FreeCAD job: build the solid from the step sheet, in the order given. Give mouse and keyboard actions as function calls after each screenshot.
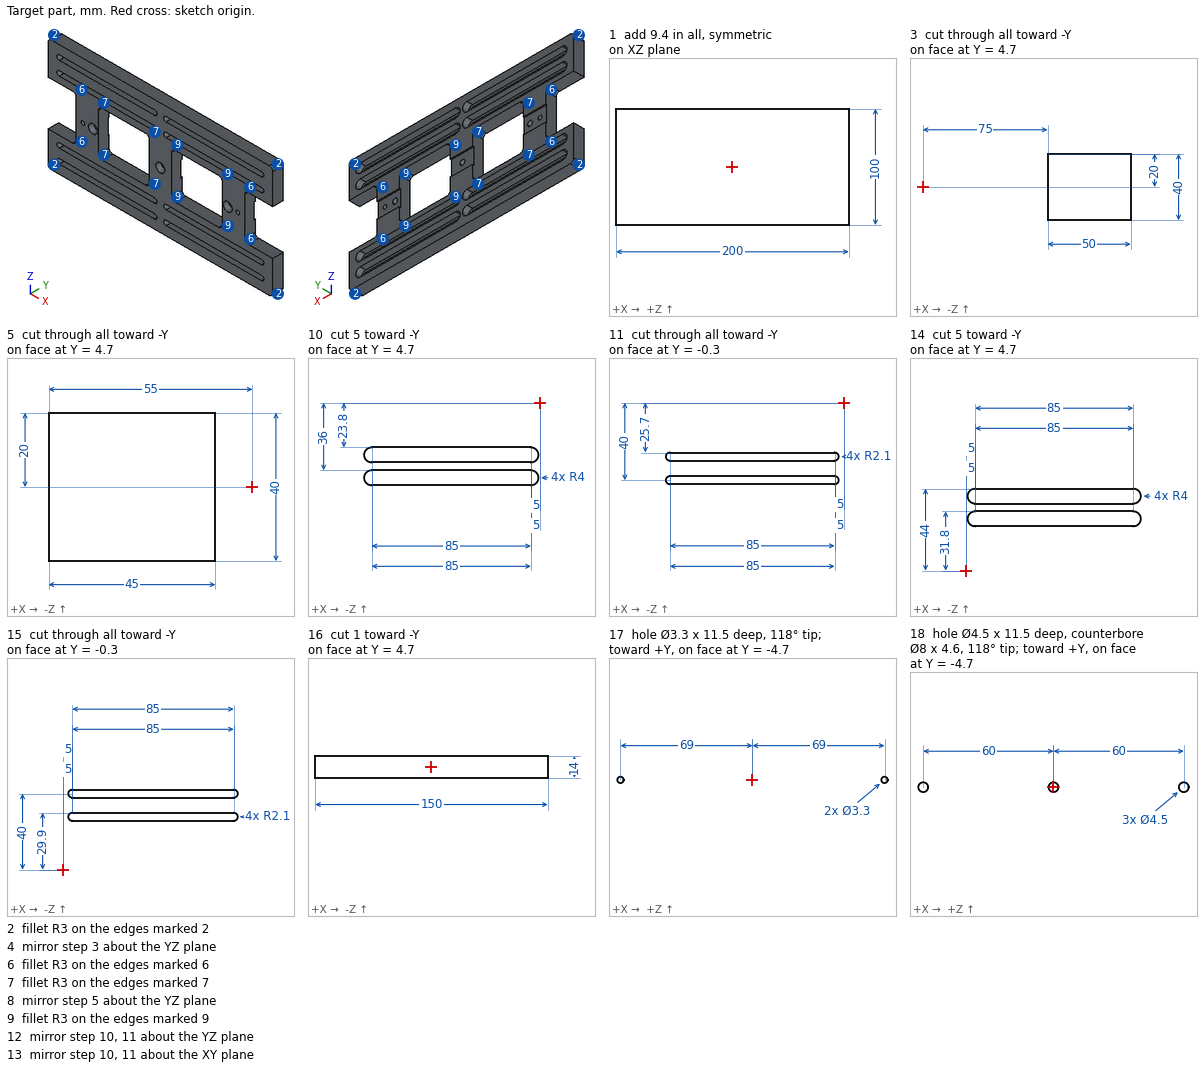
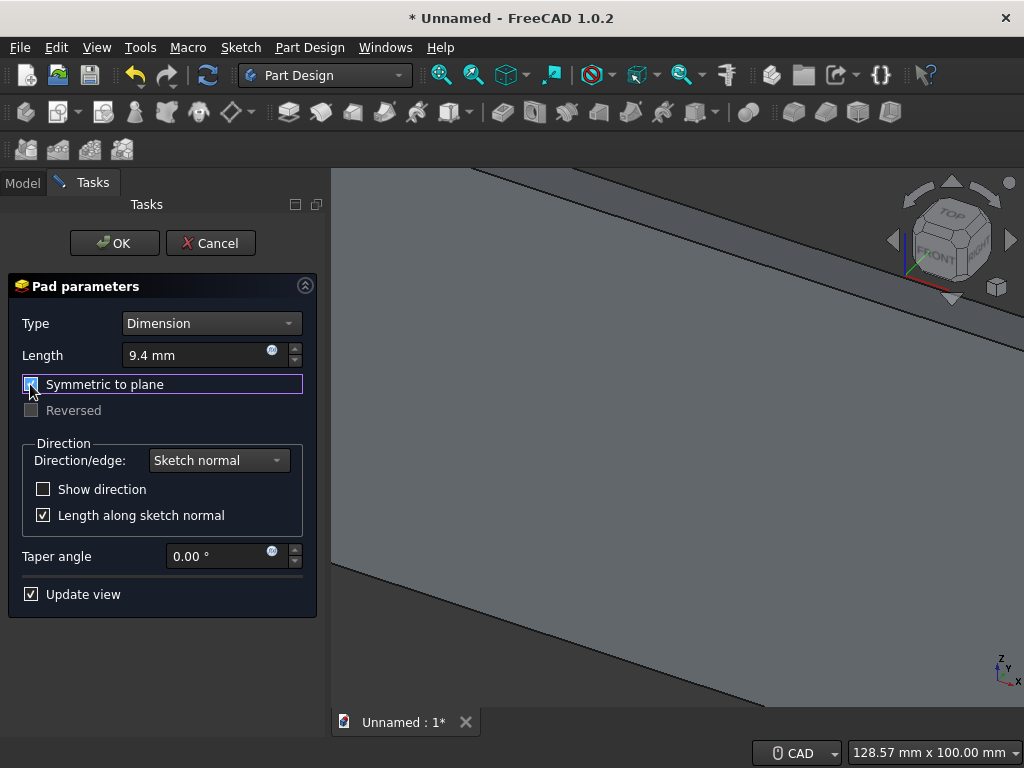
click(115, 243)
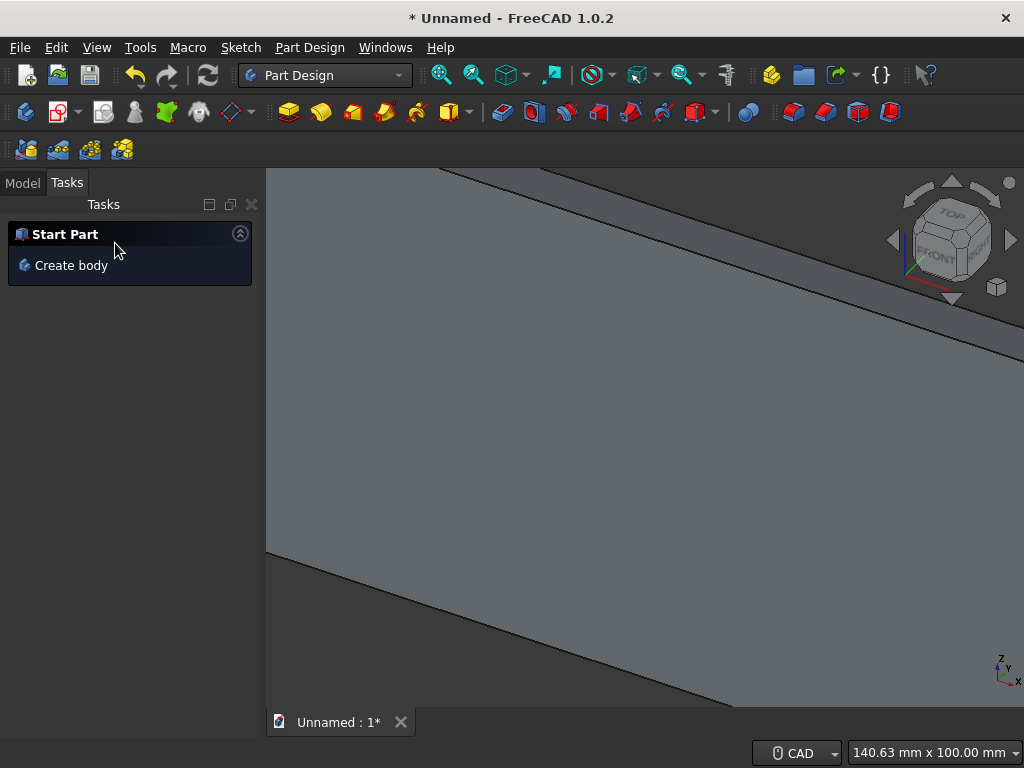
key(v)
key(f)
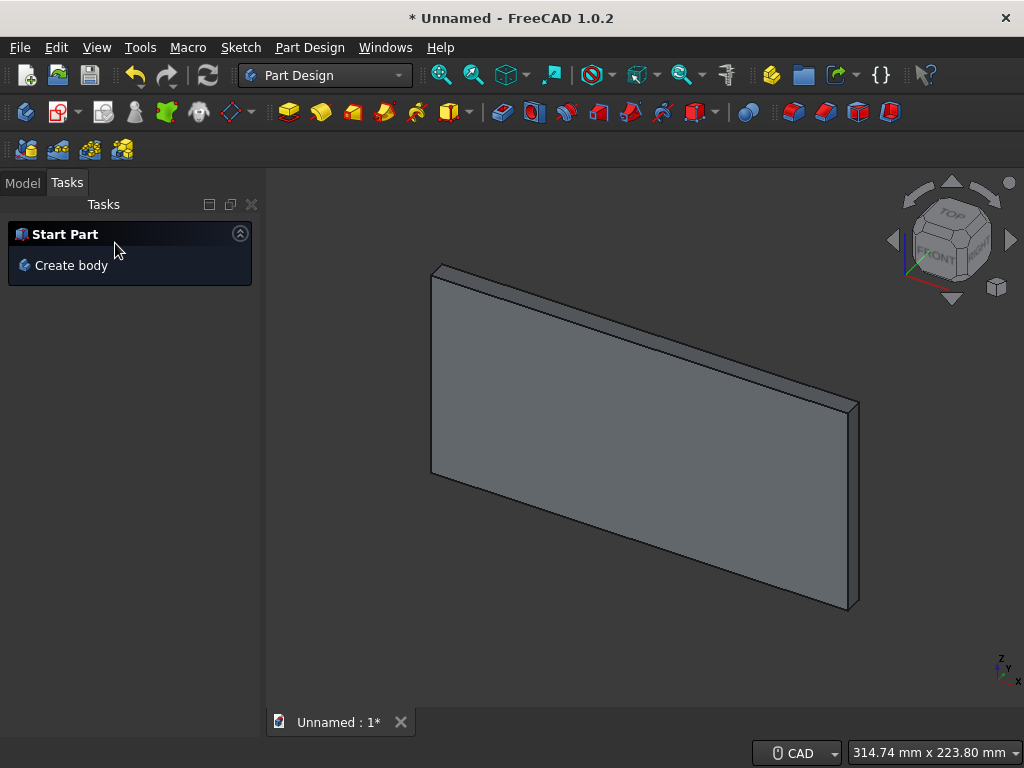
click(854, 407)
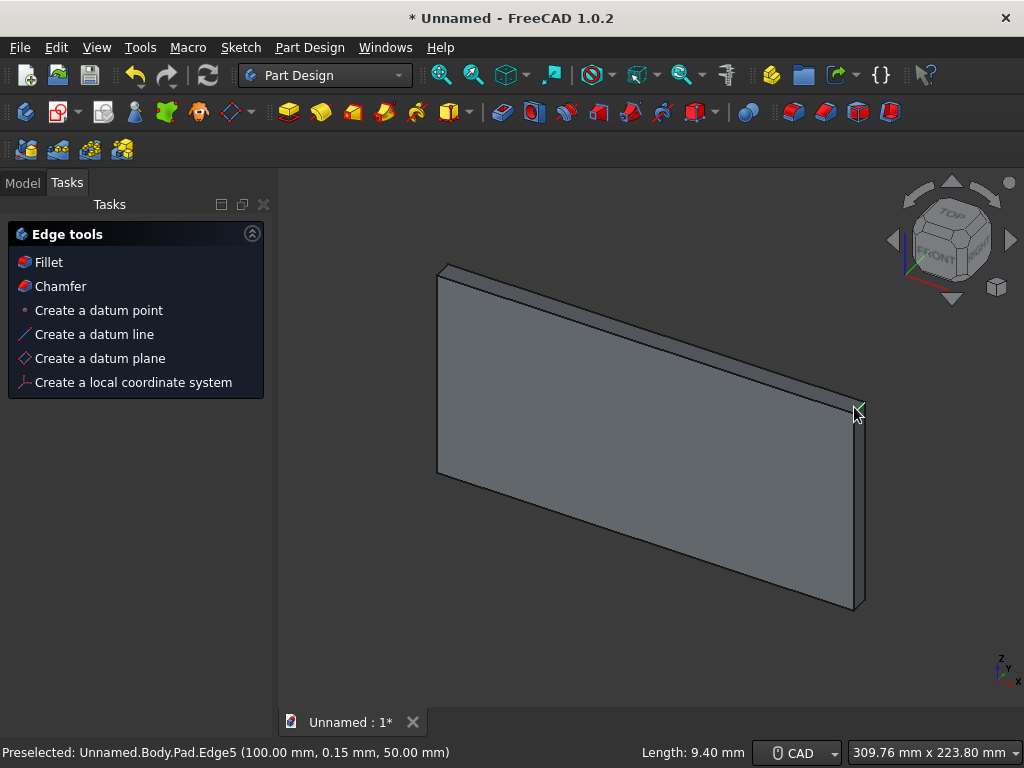
key(0)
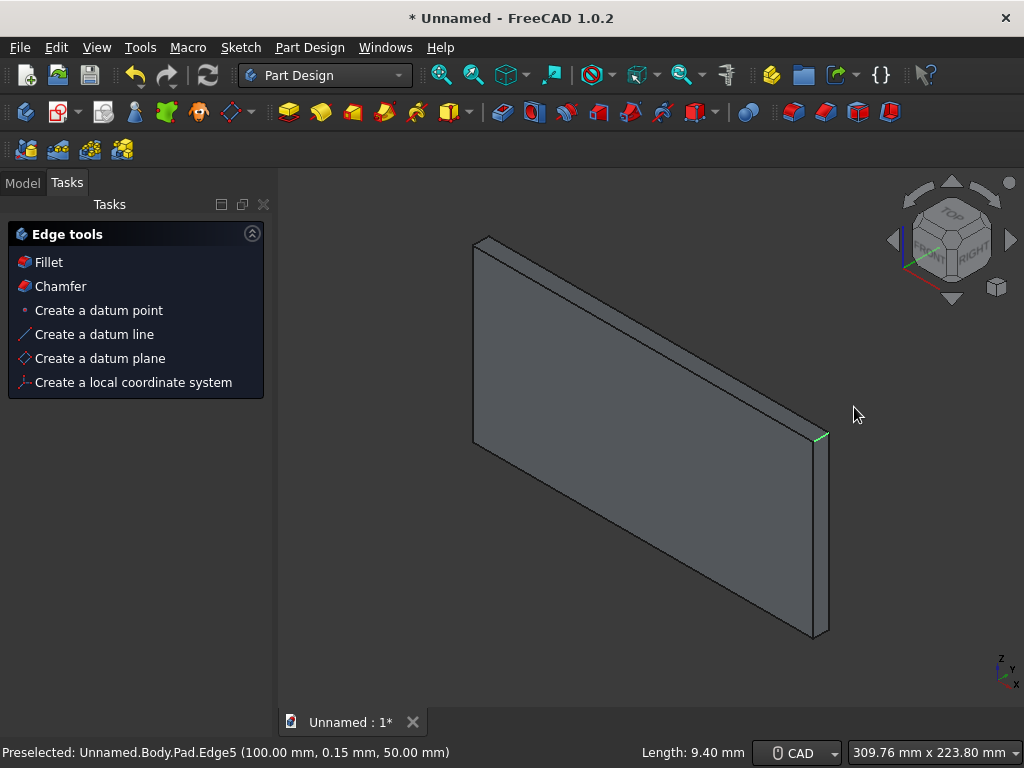
key(2)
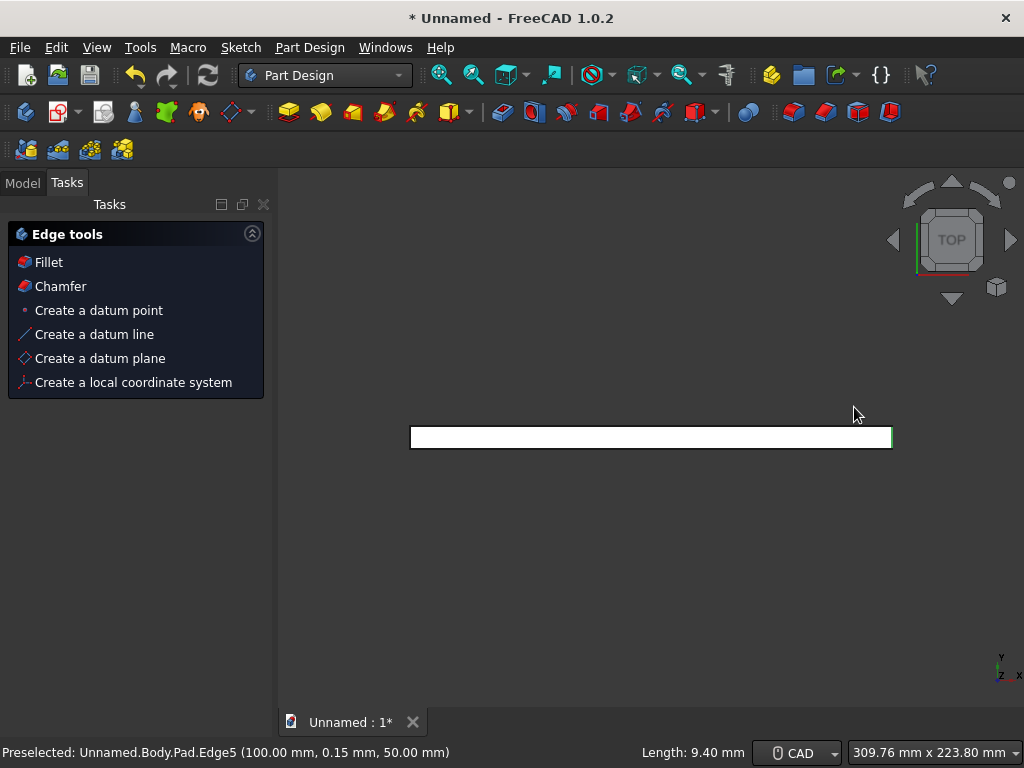
click(410, 437, ctrl)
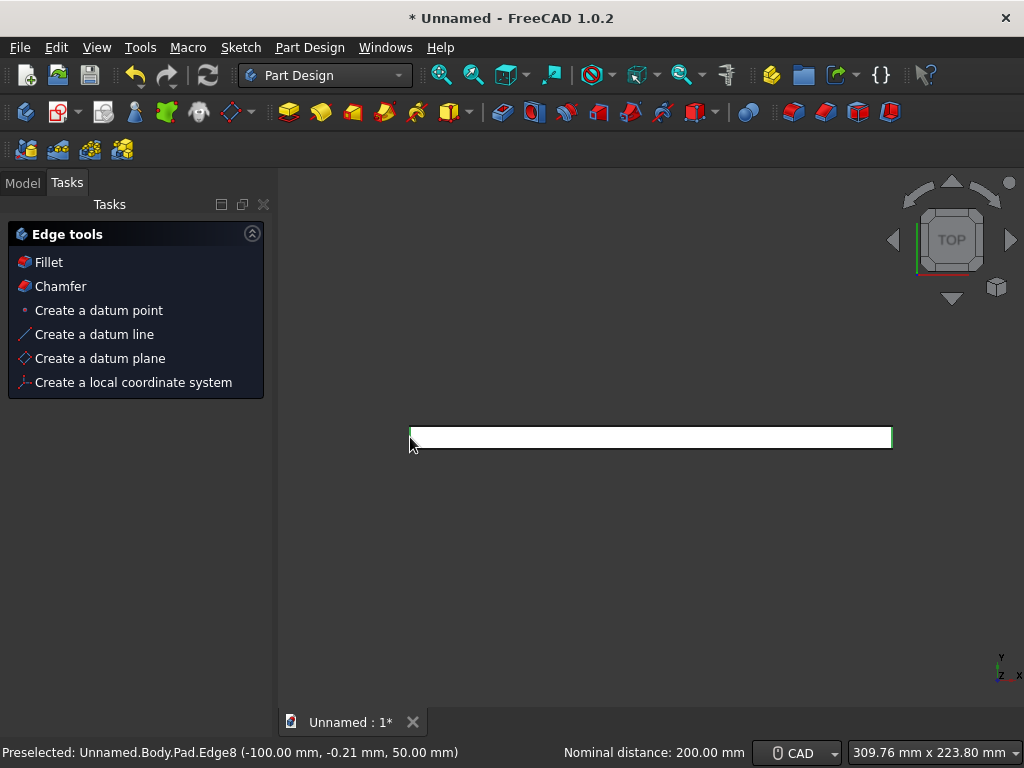
key(1)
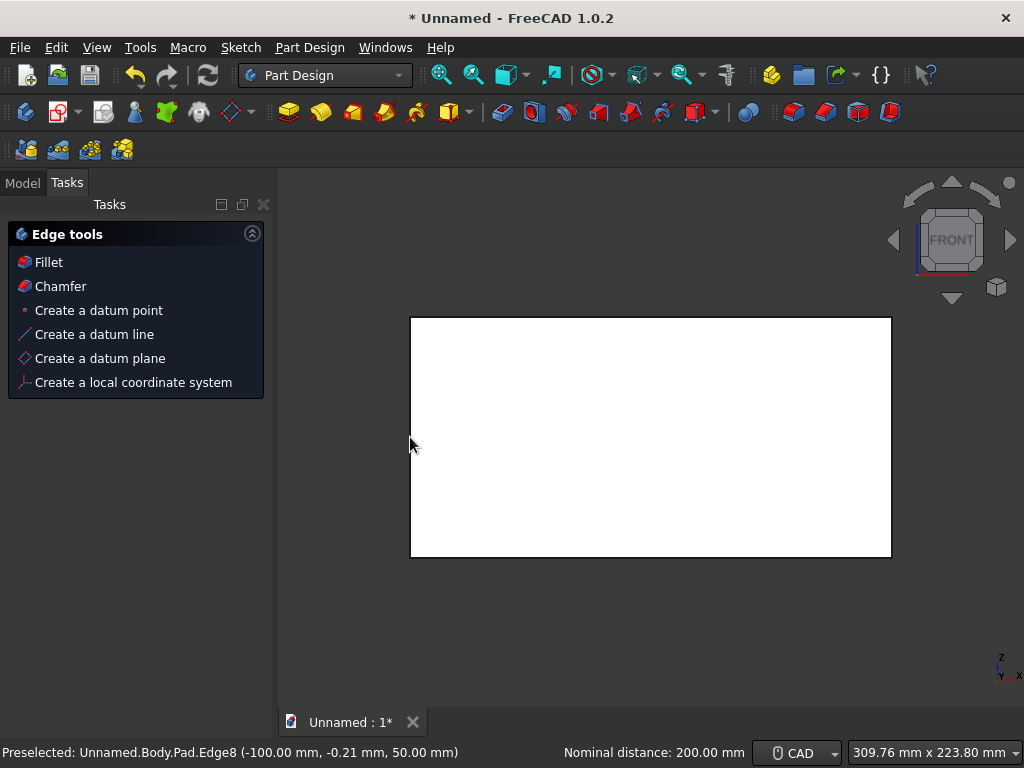
key(3)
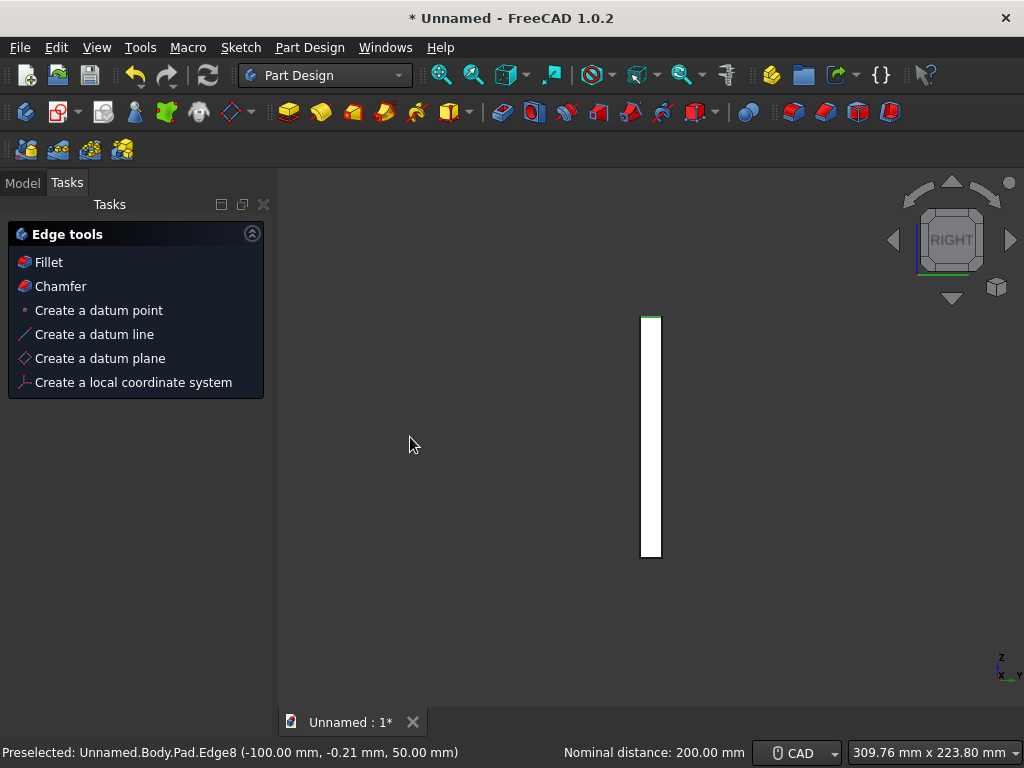
click(442, 76)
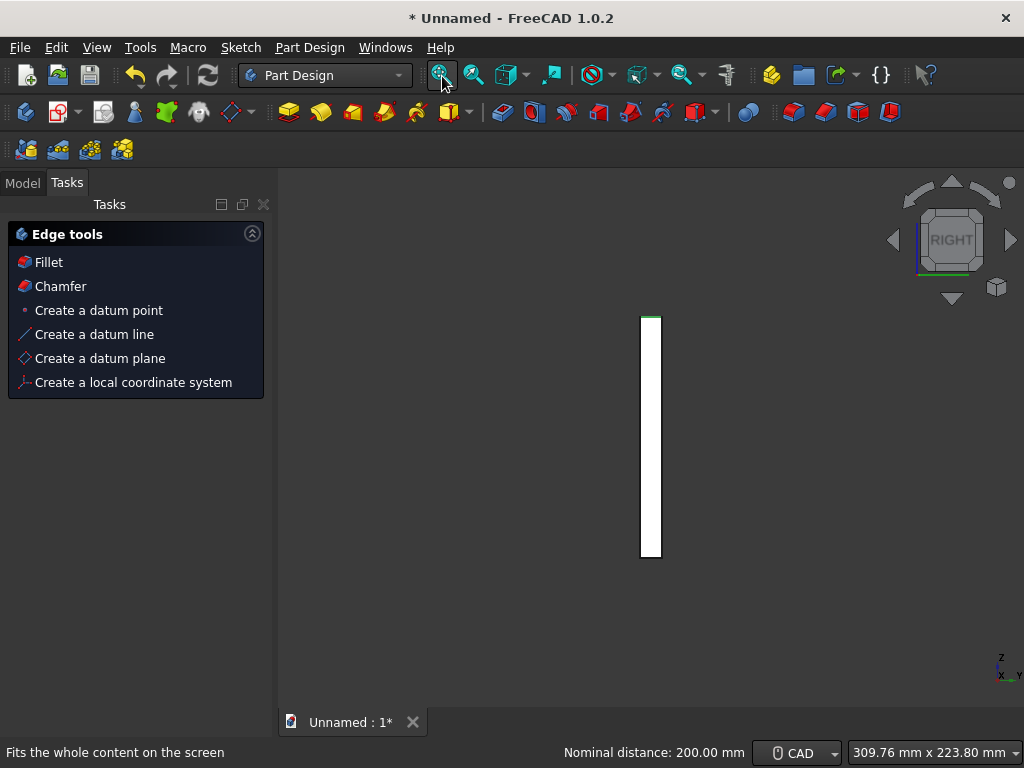
click(651, 557, ctrl)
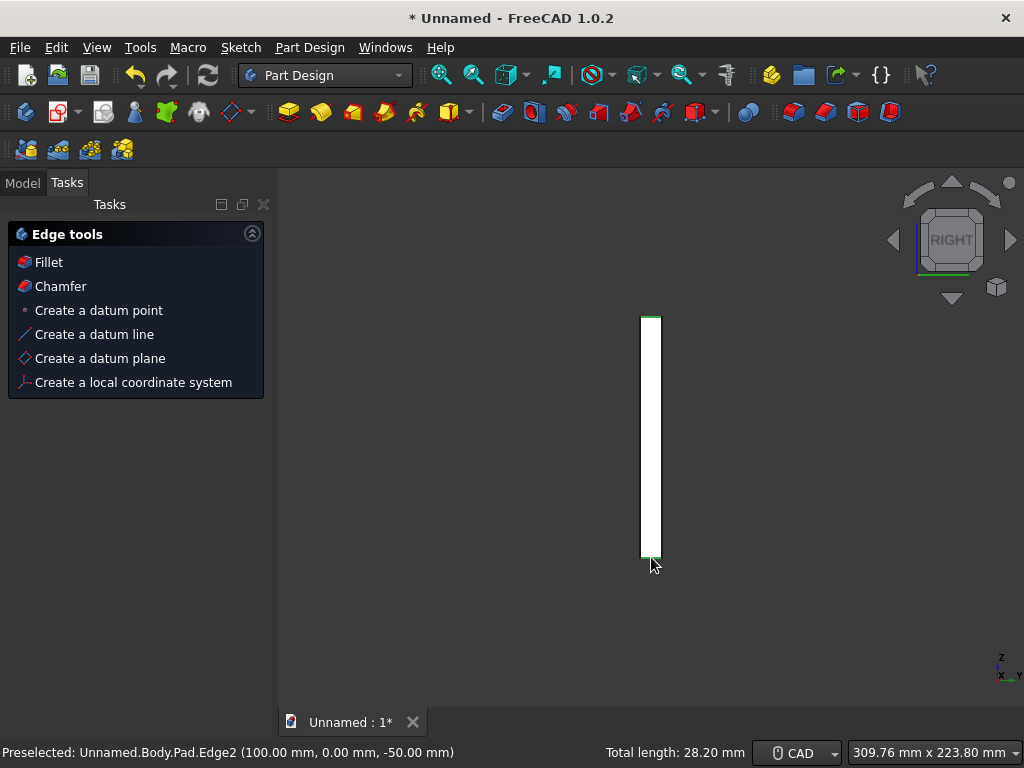
key(5)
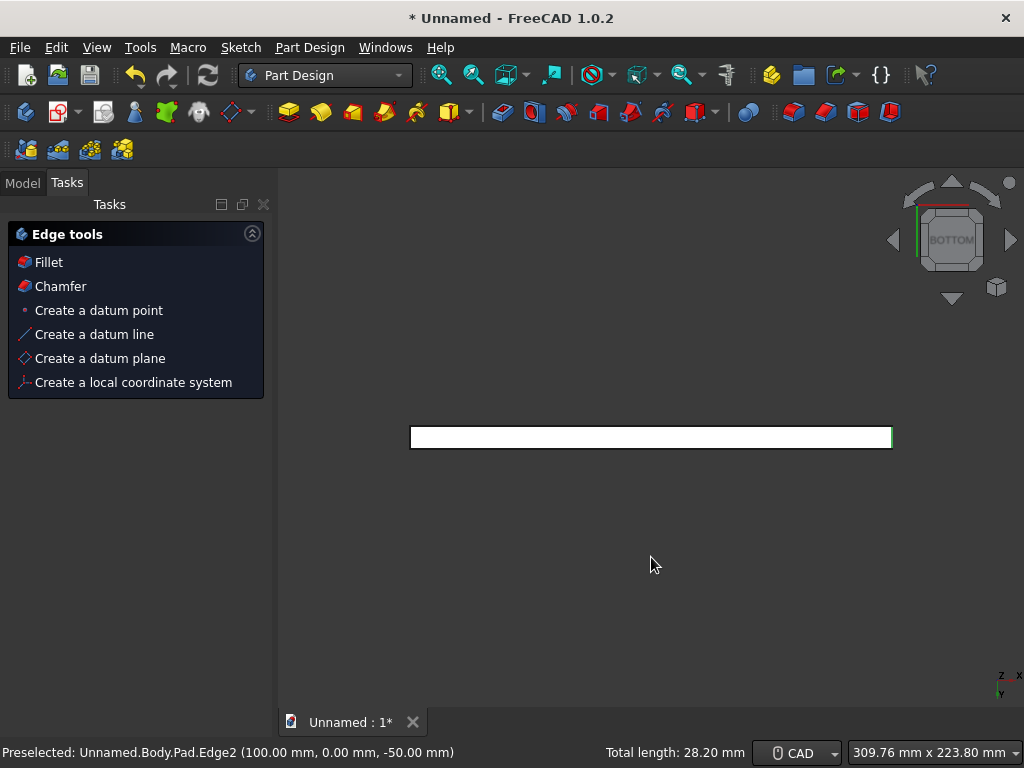
click(410, 436, ctrl)